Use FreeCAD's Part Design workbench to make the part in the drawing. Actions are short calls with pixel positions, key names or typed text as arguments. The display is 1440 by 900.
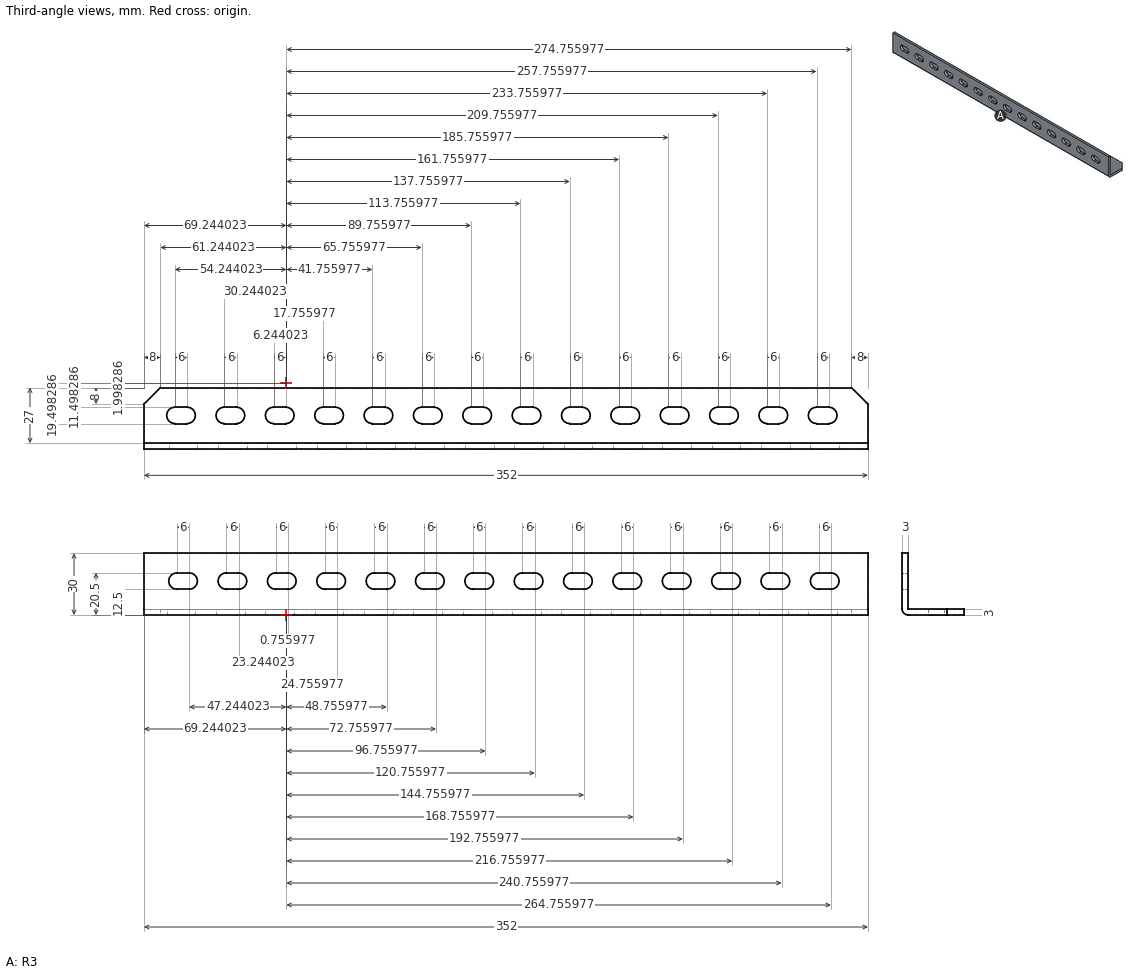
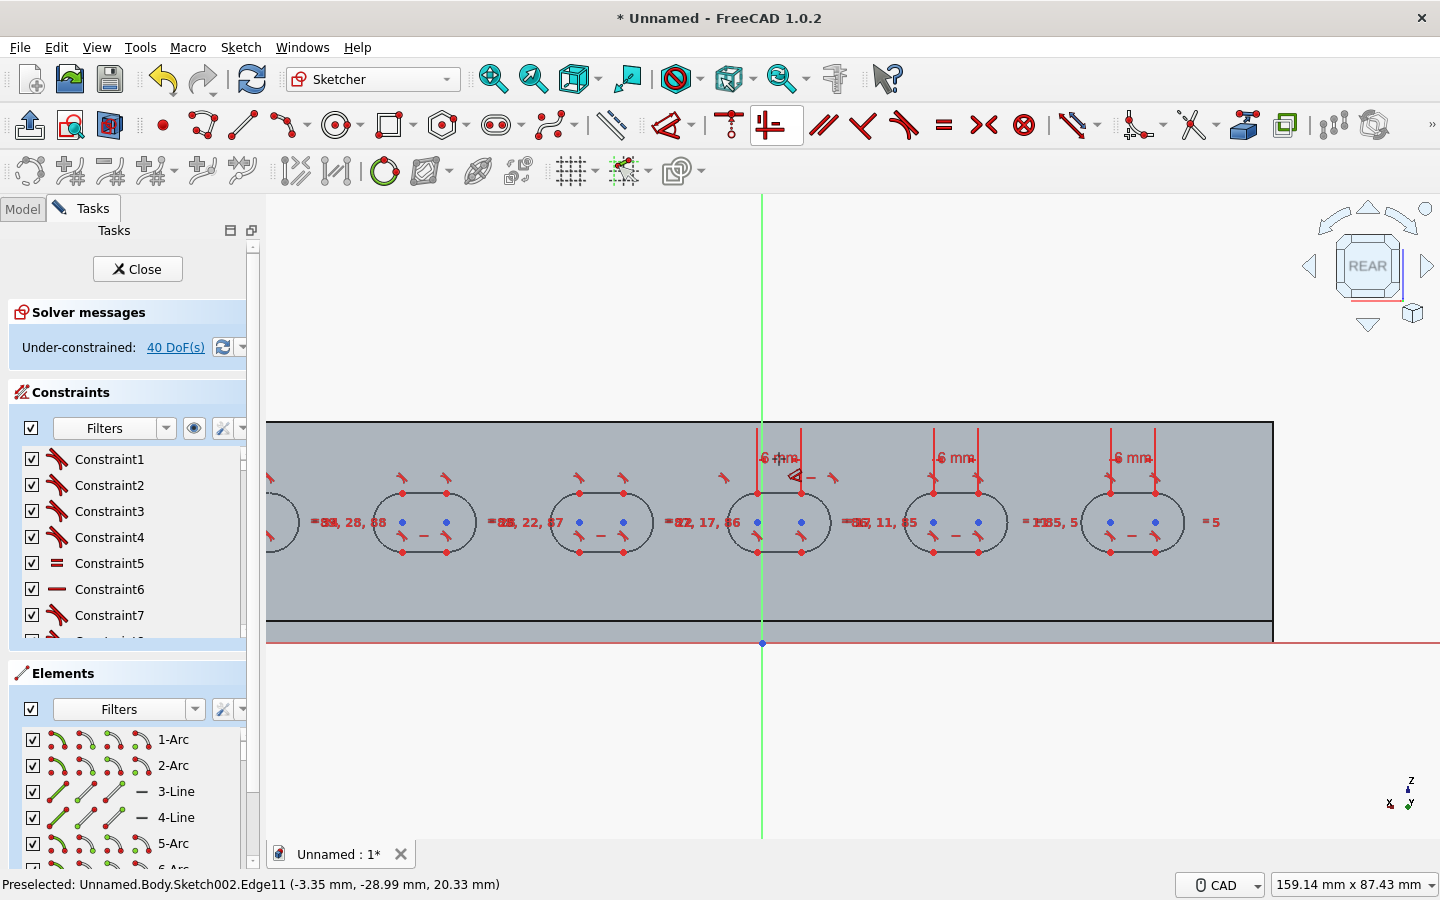
click(593, 493)
click(602, 459)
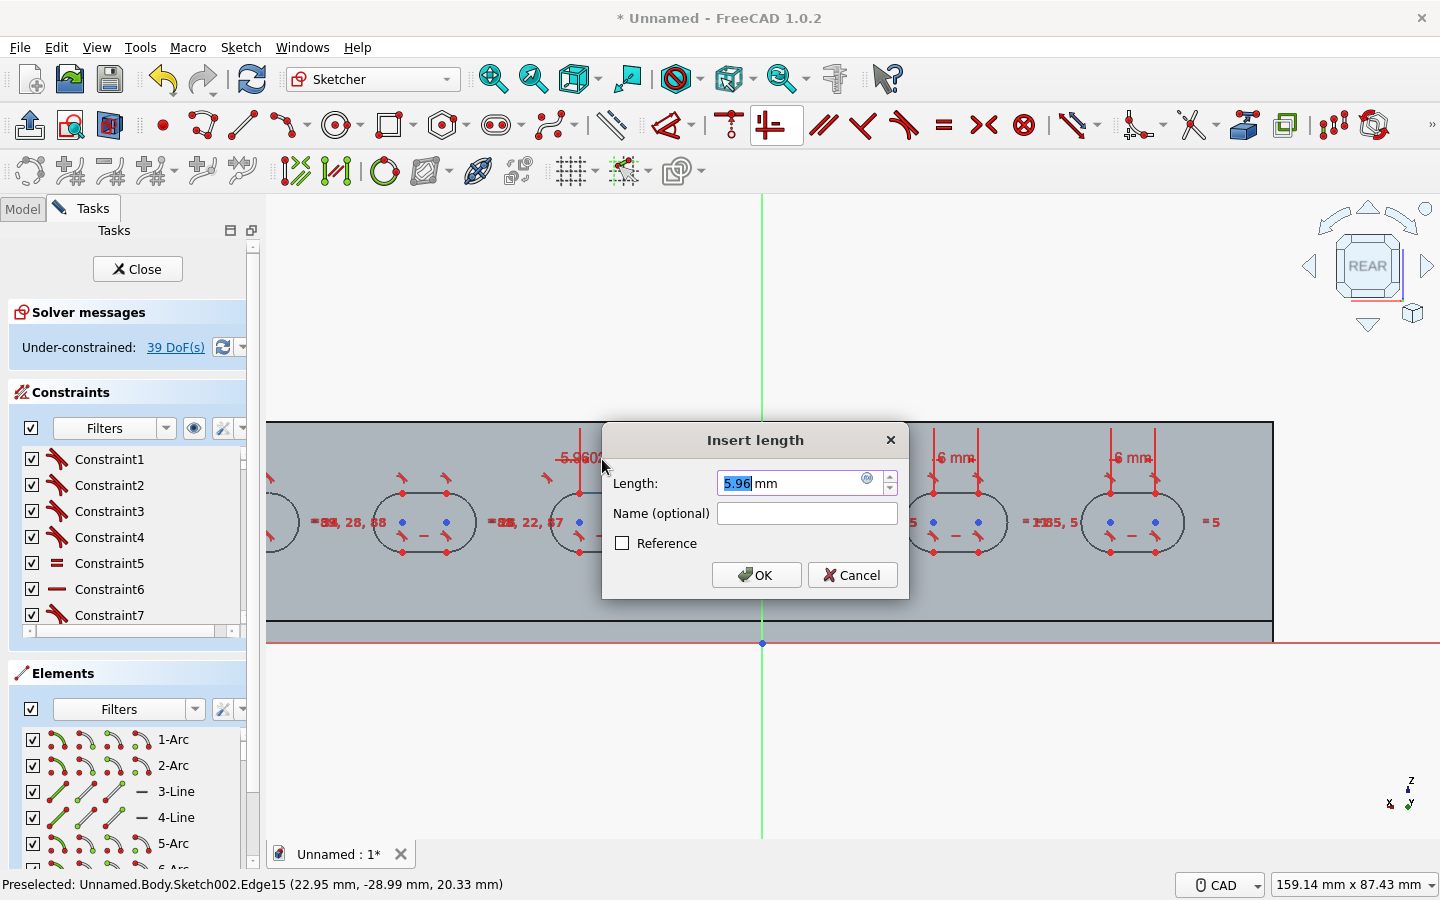
text(6)
key(Return)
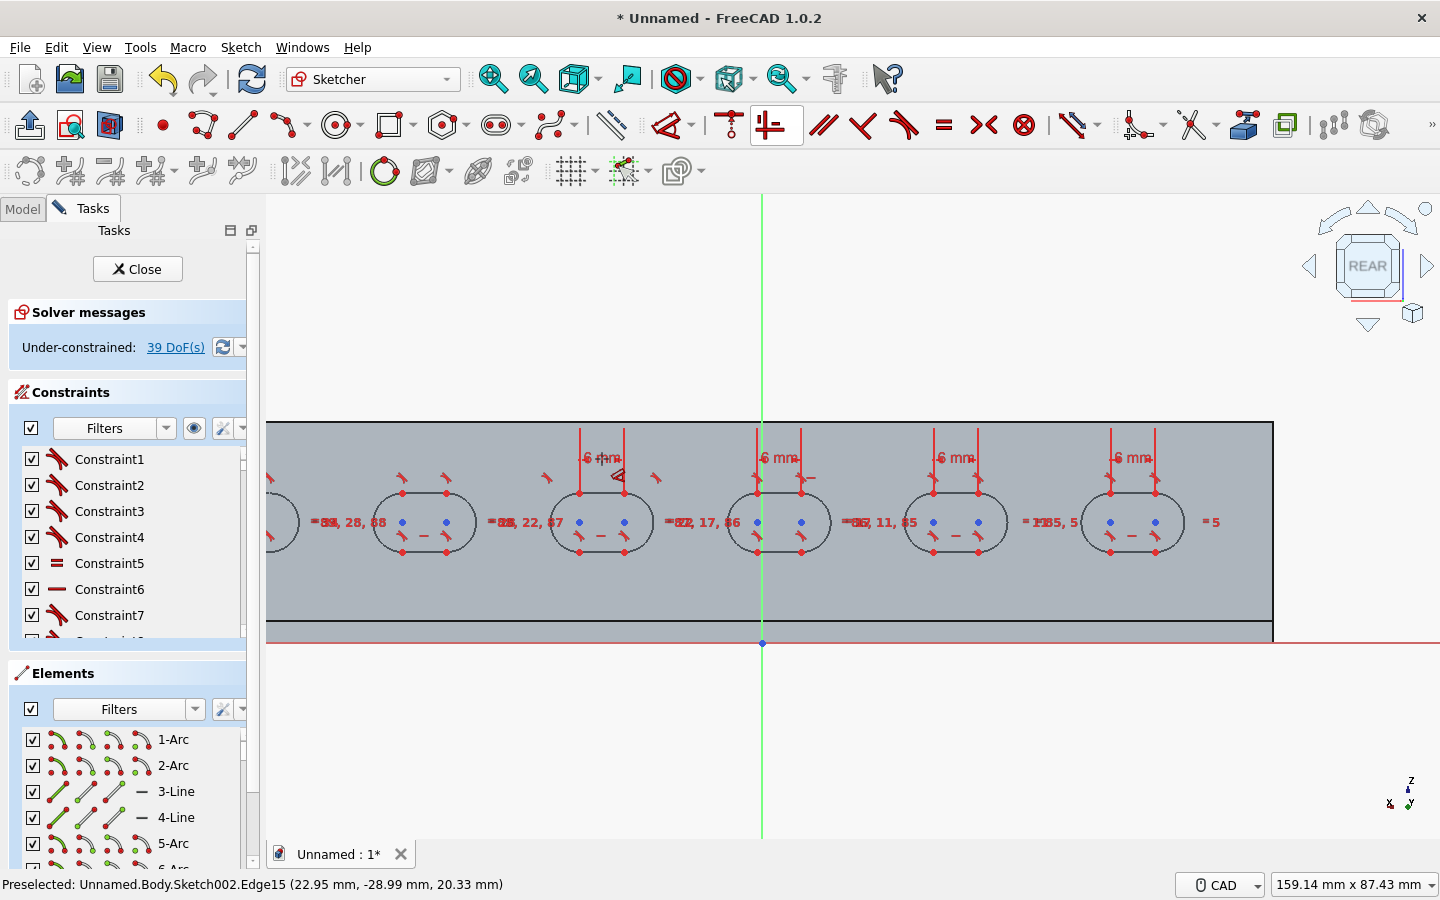
click(416, 493)
click(425, 459)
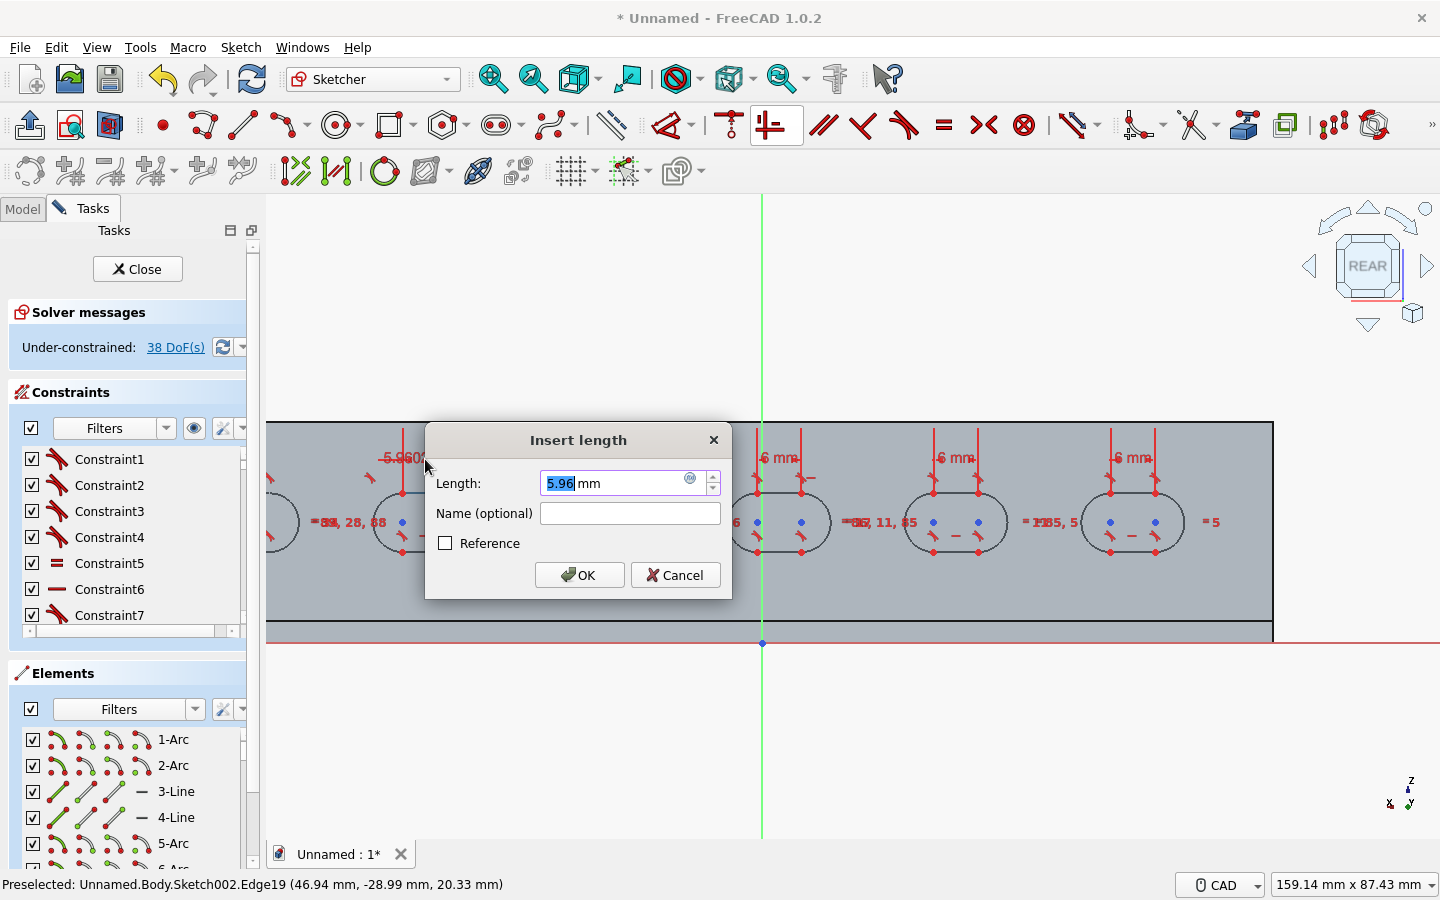
text(6)
key(Return)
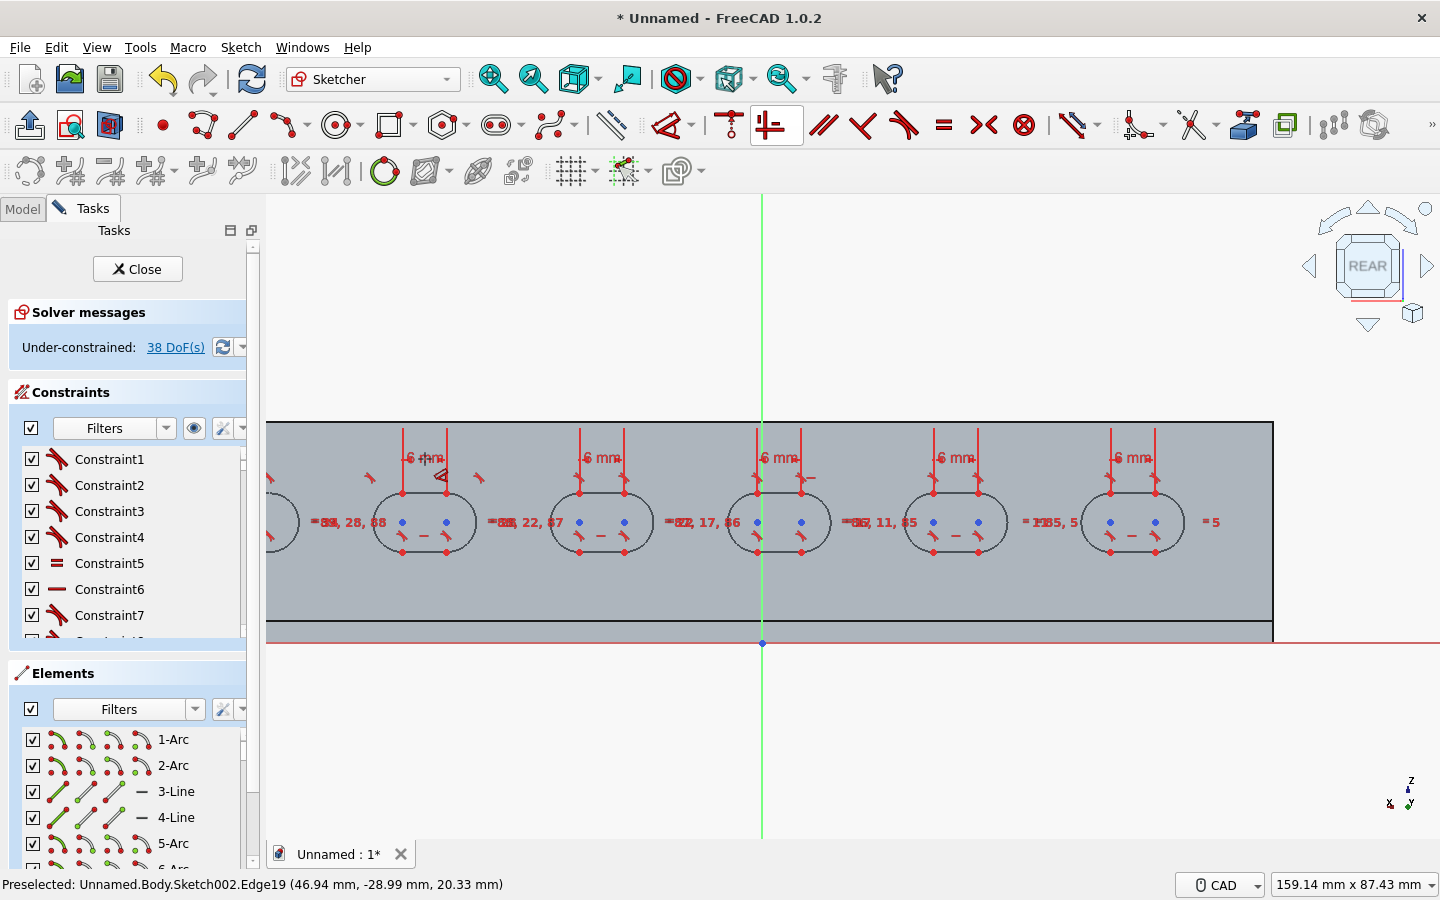
scroll(1130, 494, down, 6)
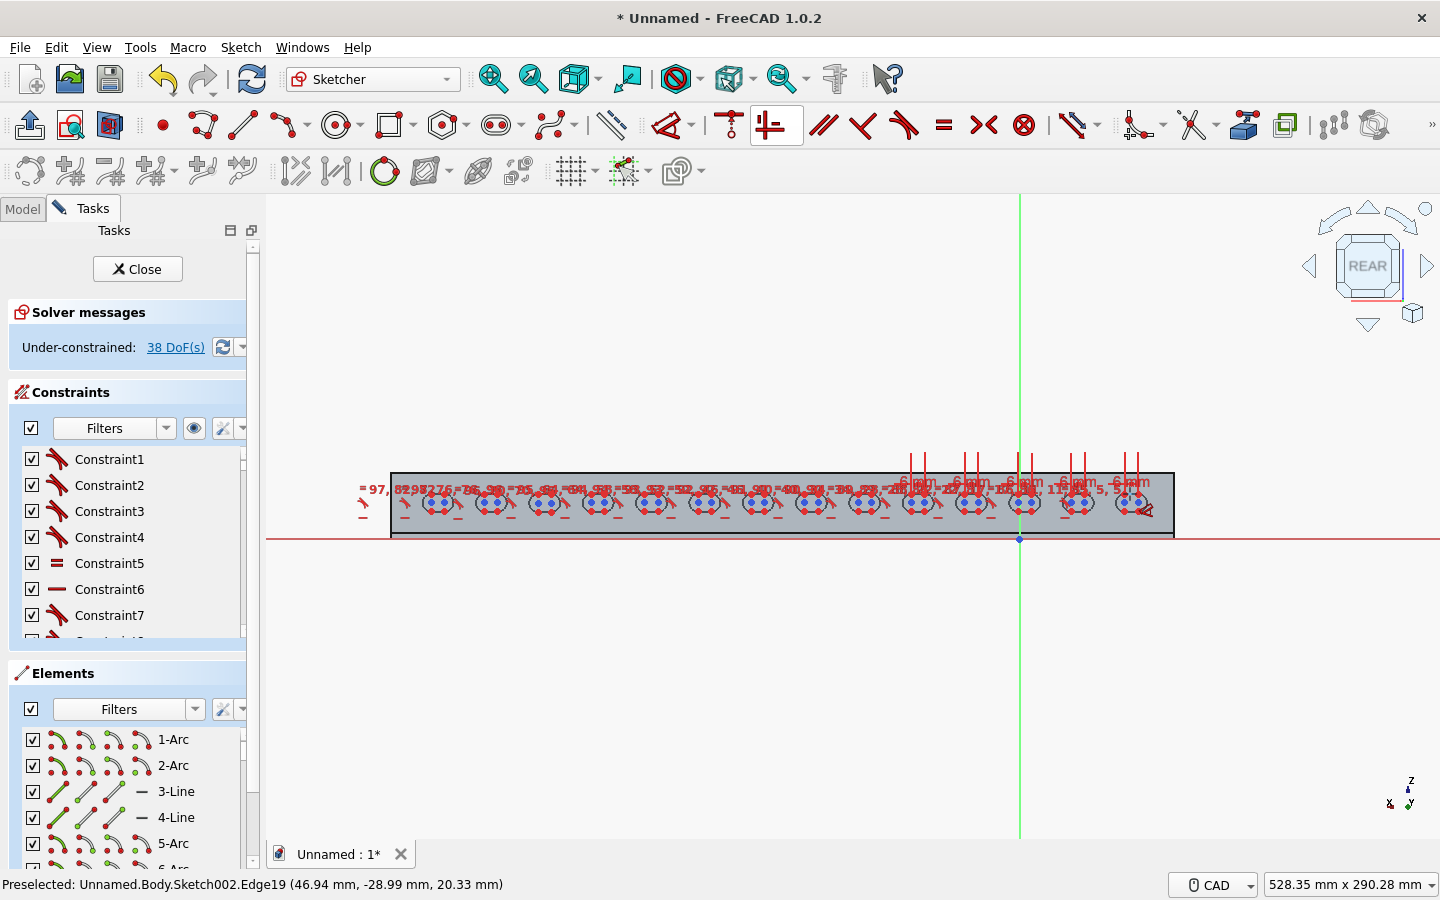
scroll(862, 494, up, 7)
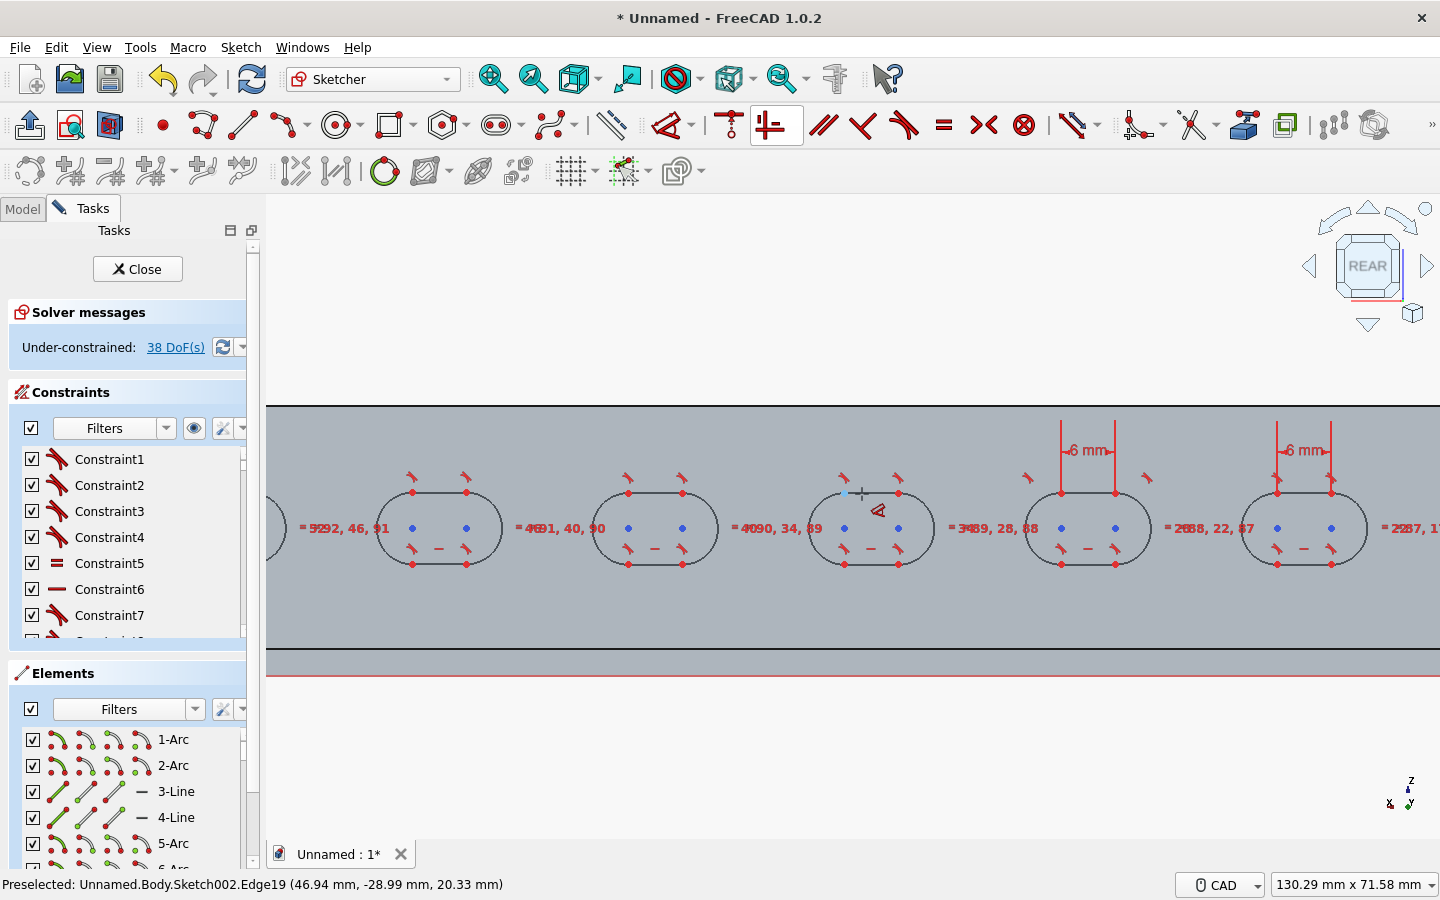
click(861, 493)
click(872, 459)